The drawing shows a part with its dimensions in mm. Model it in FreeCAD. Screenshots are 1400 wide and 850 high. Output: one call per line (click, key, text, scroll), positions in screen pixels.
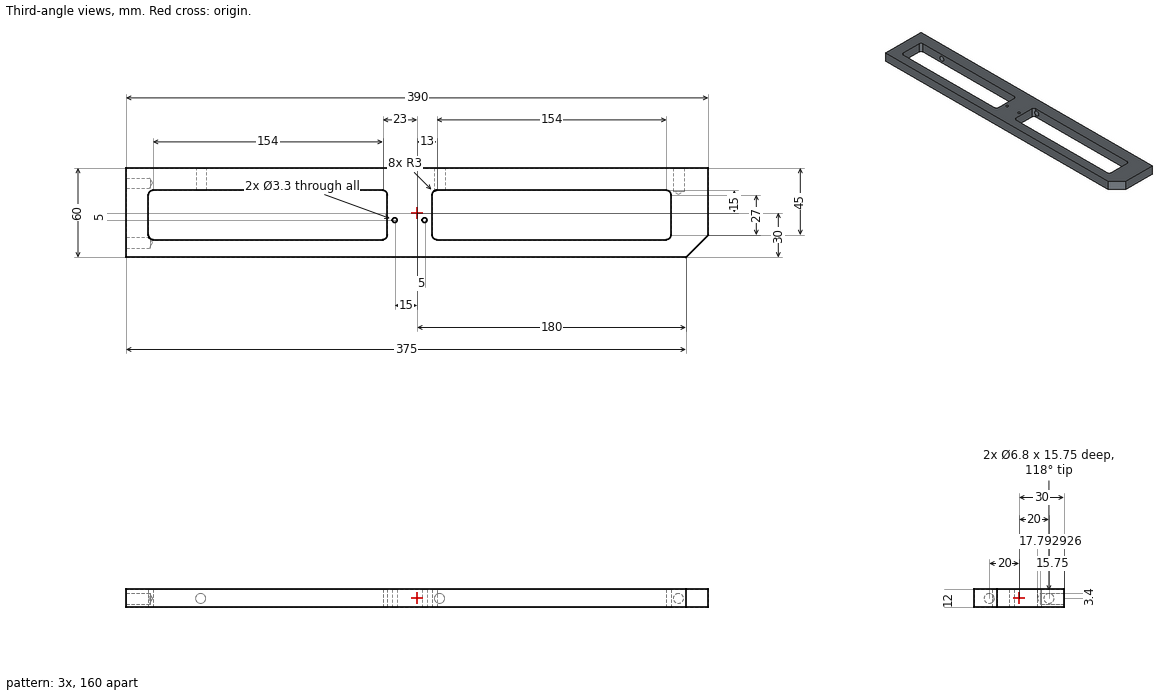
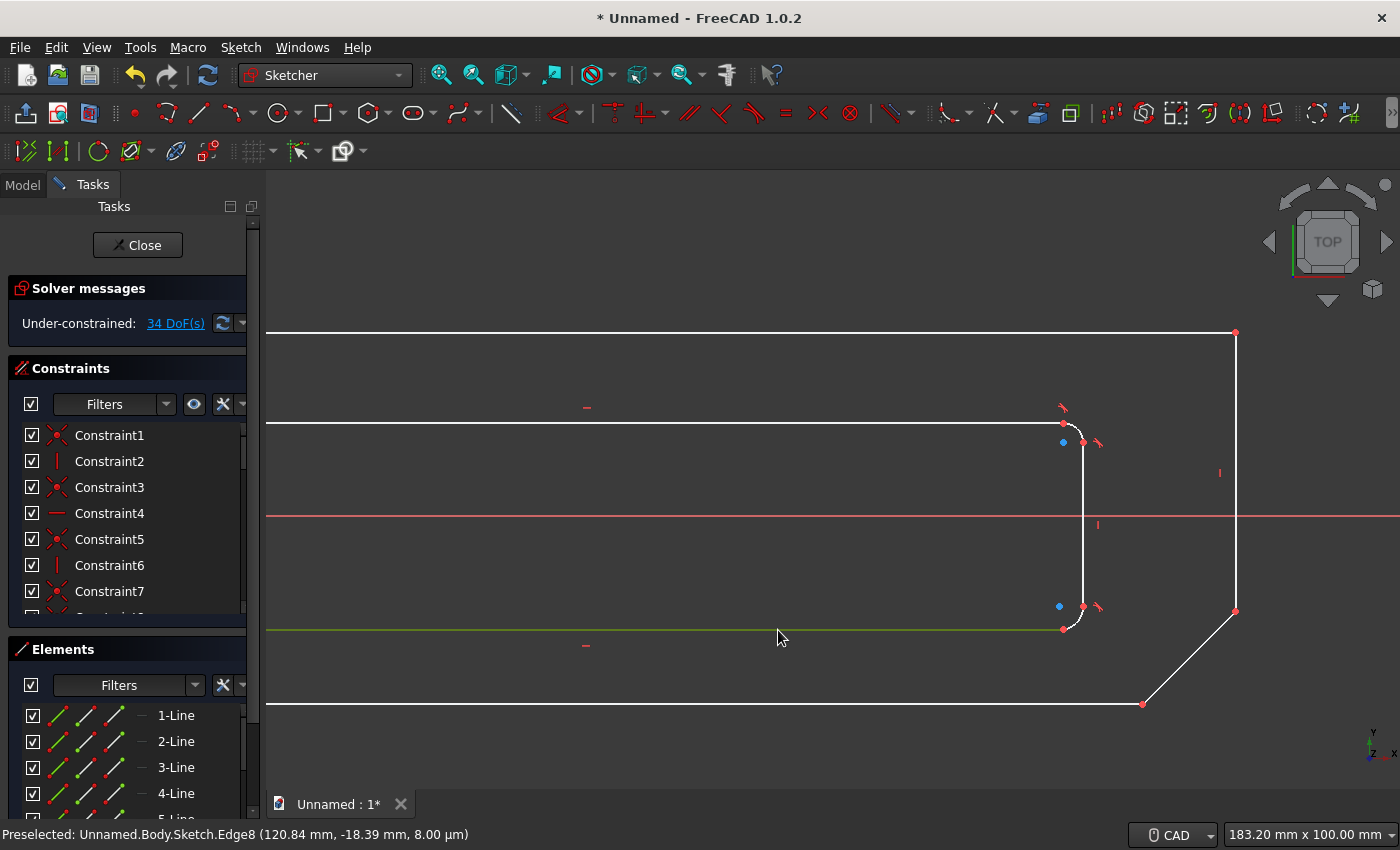
scroll(1073, 626, up, 2)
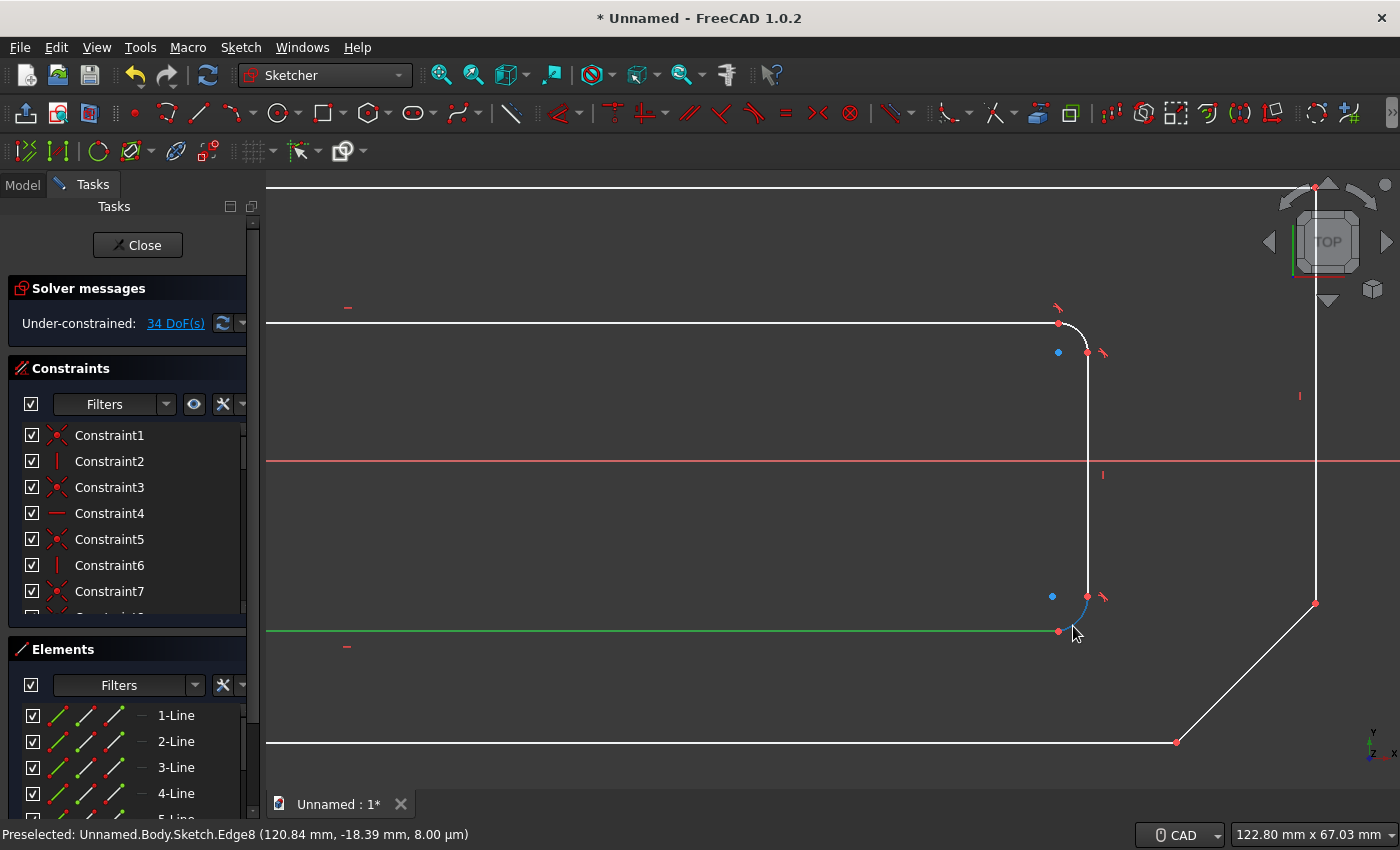
click(1072, 626)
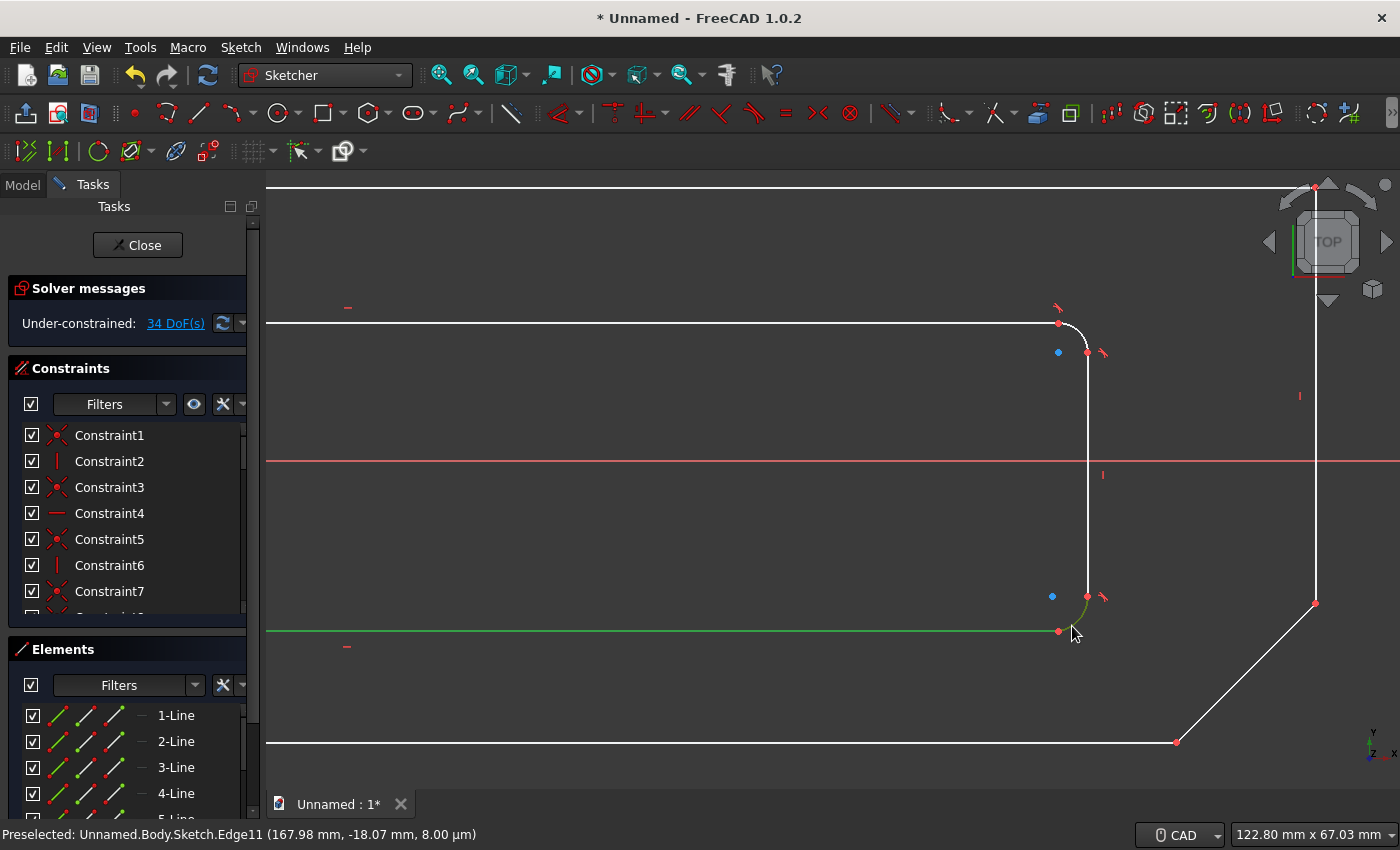
click(754, 114)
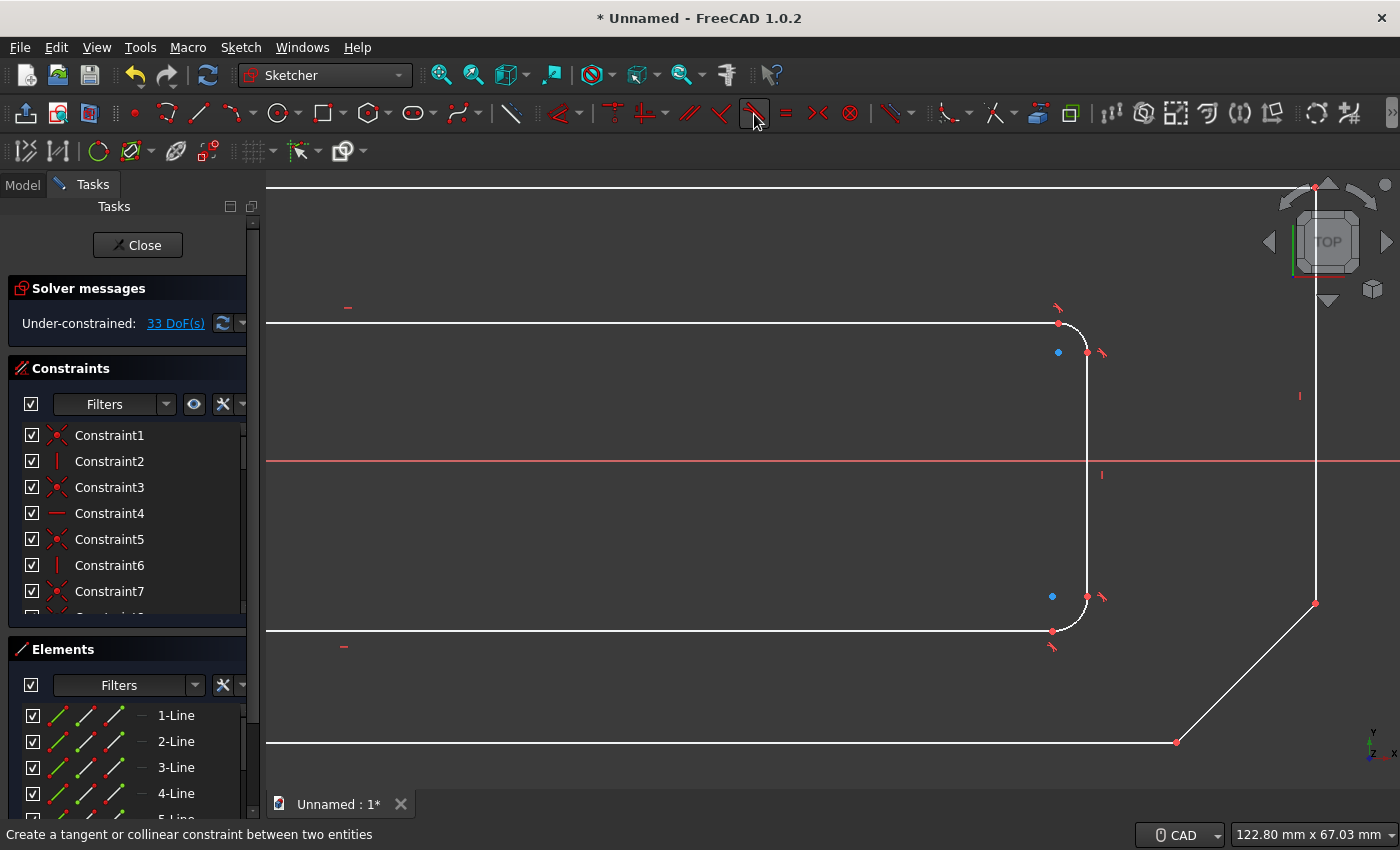
scroll(1080, 484, down, 8)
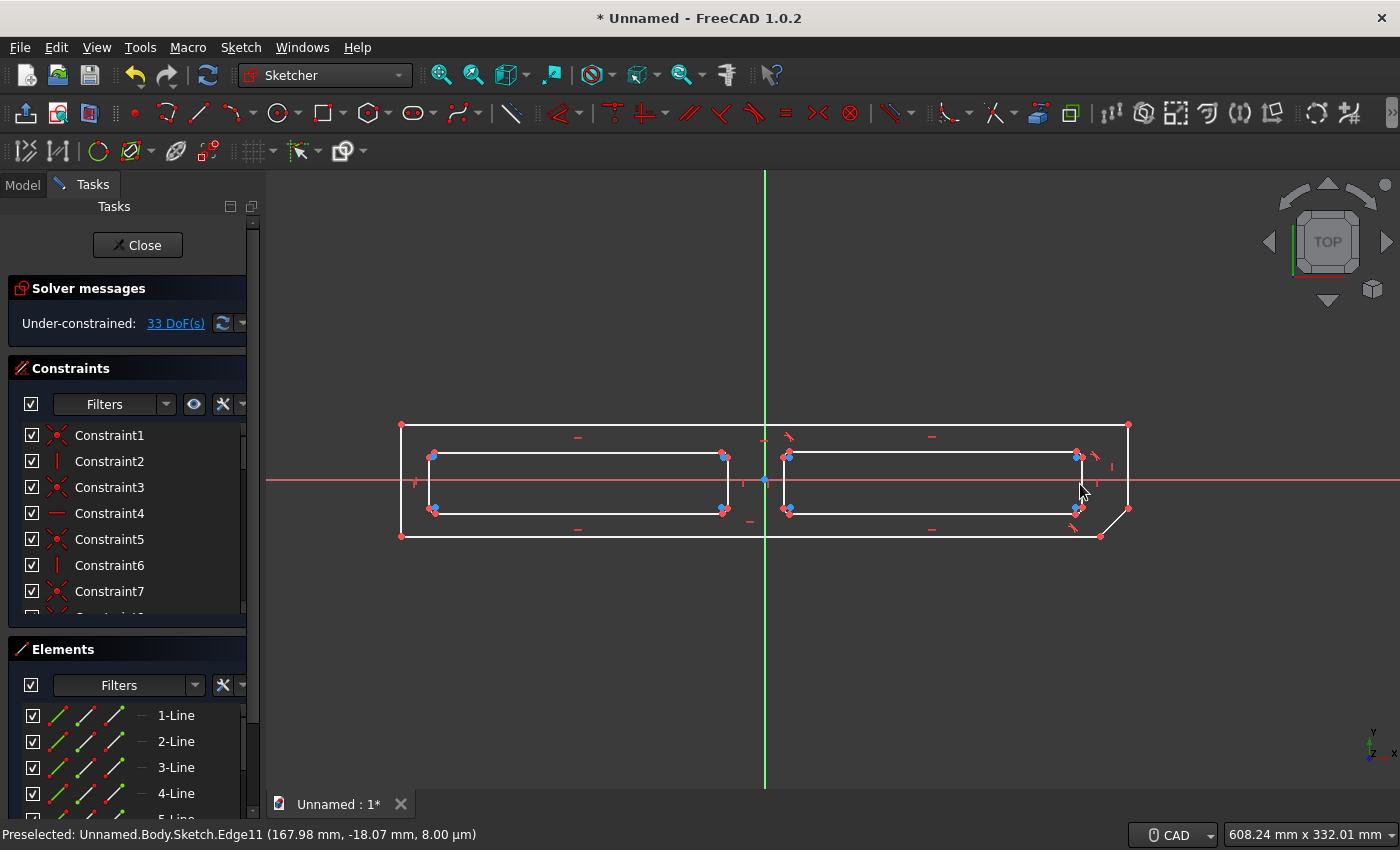
click(989, 514)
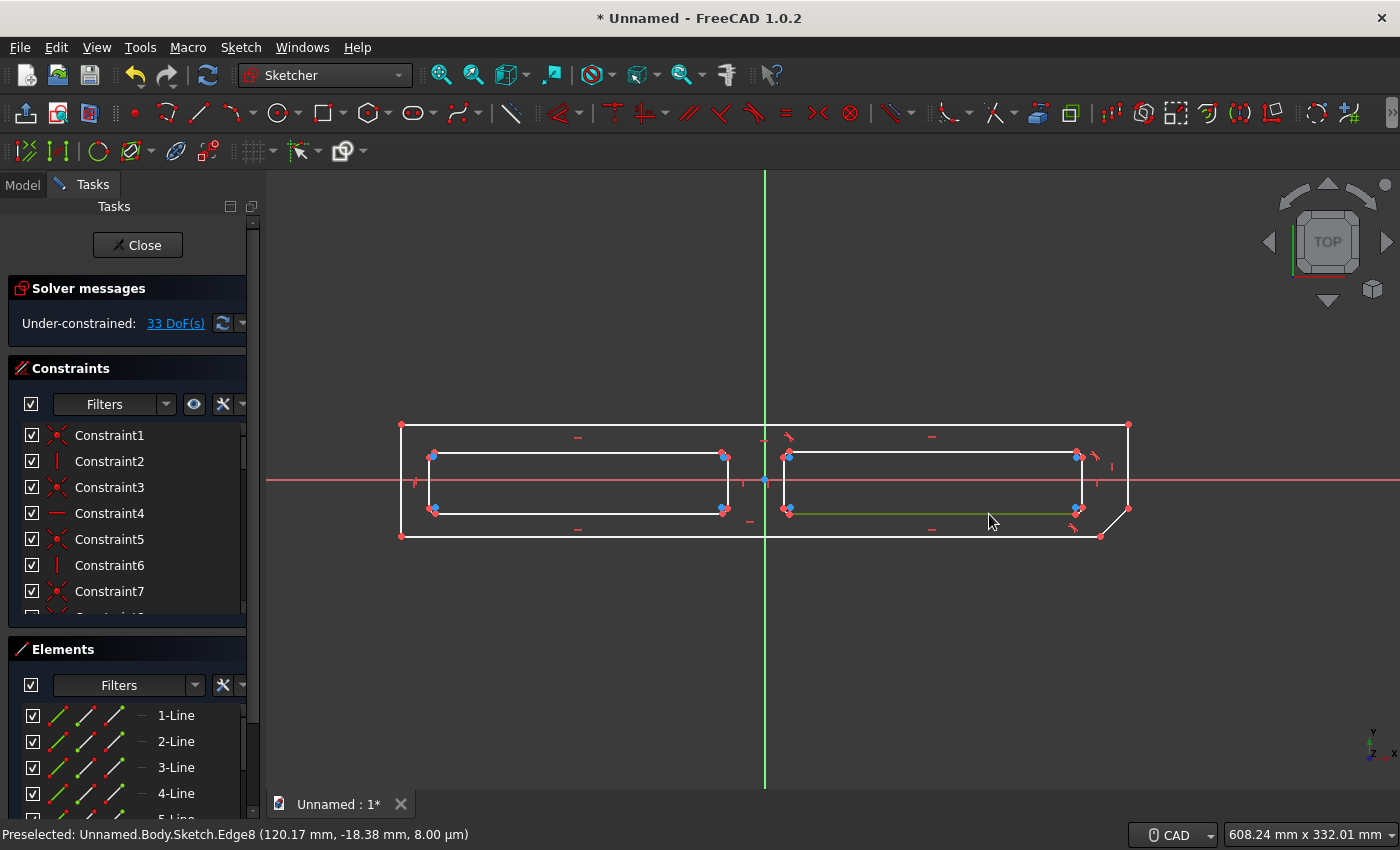
scroll(785, 512, up, 6)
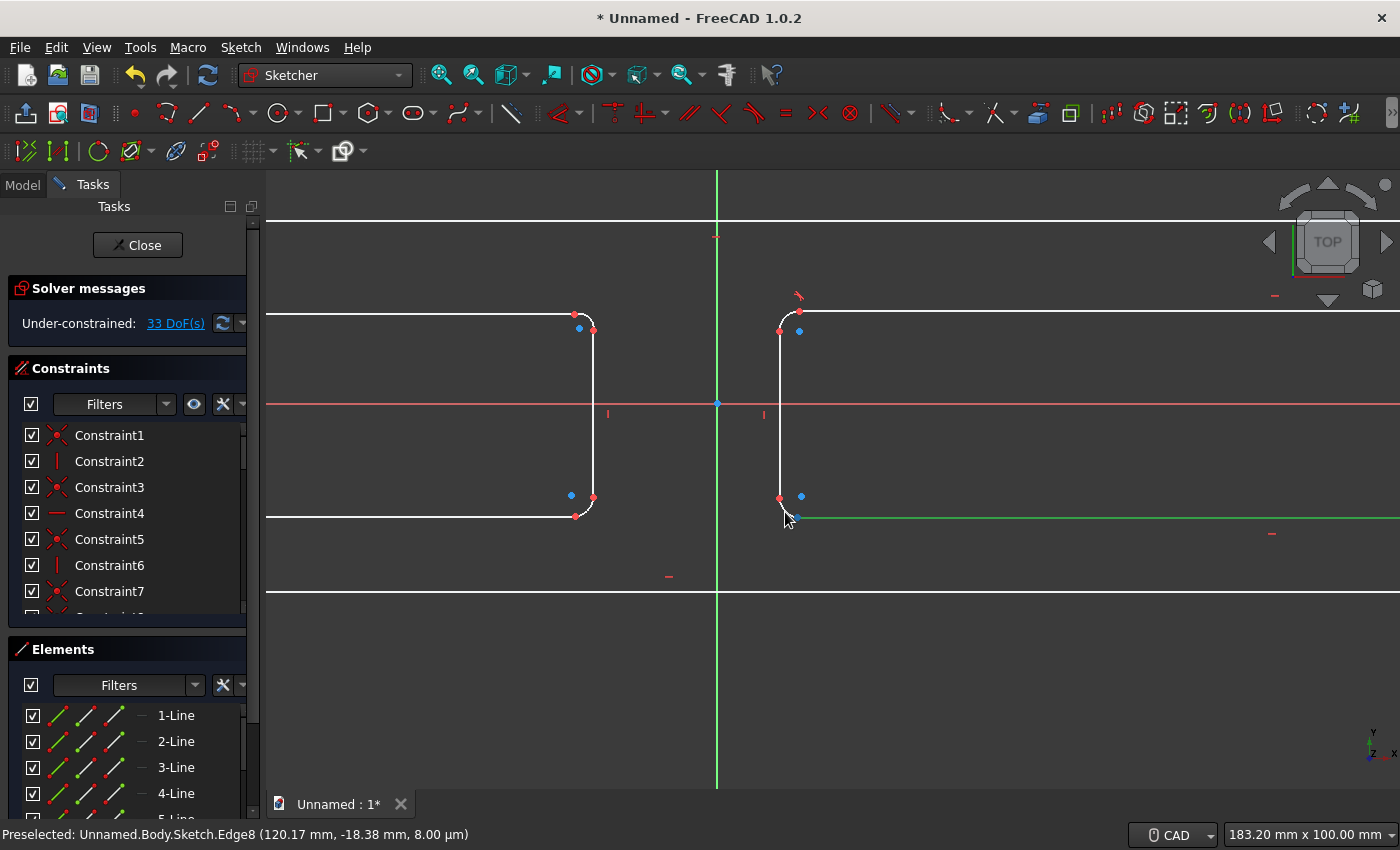
click(785, 511)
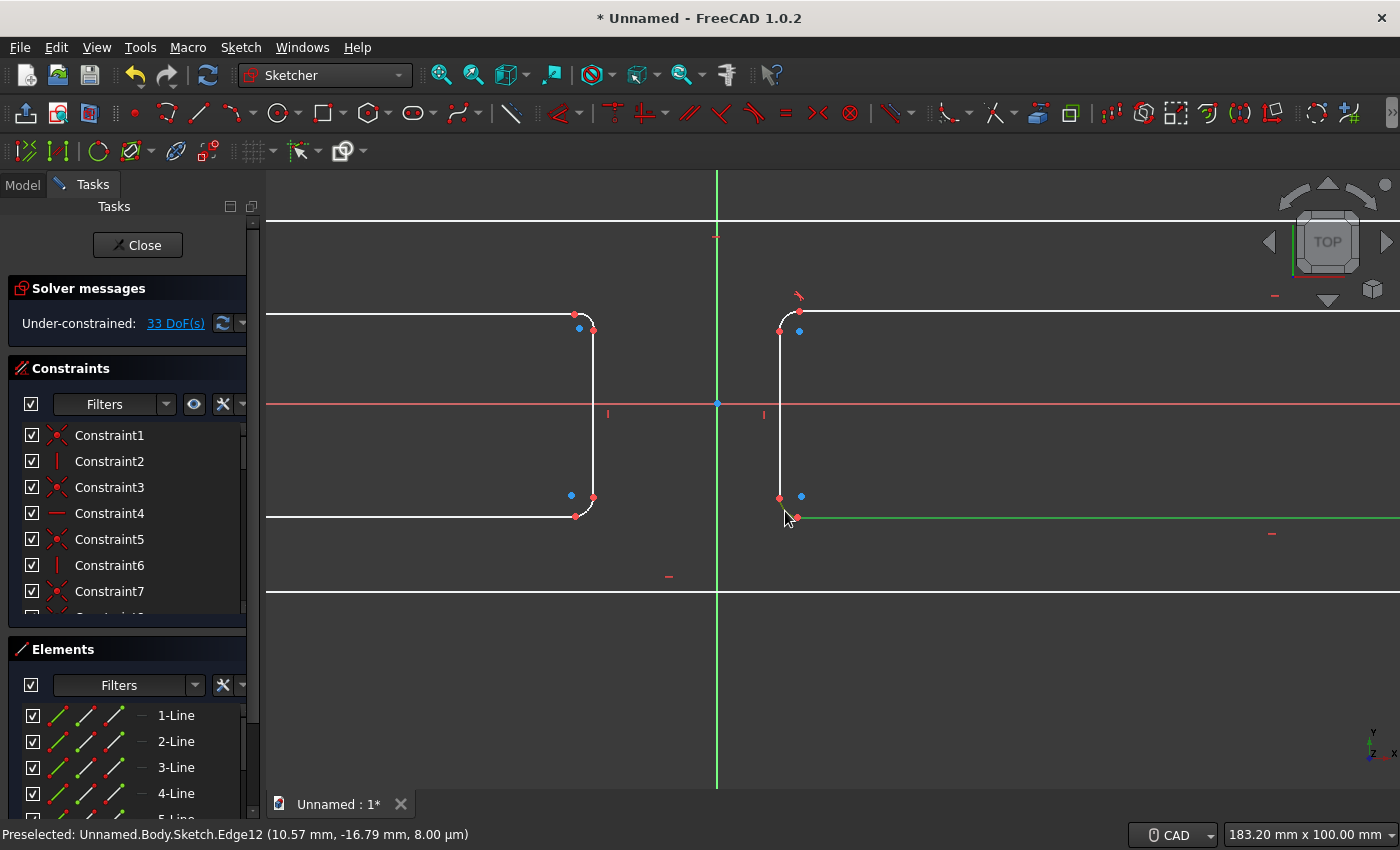
click(754, 114)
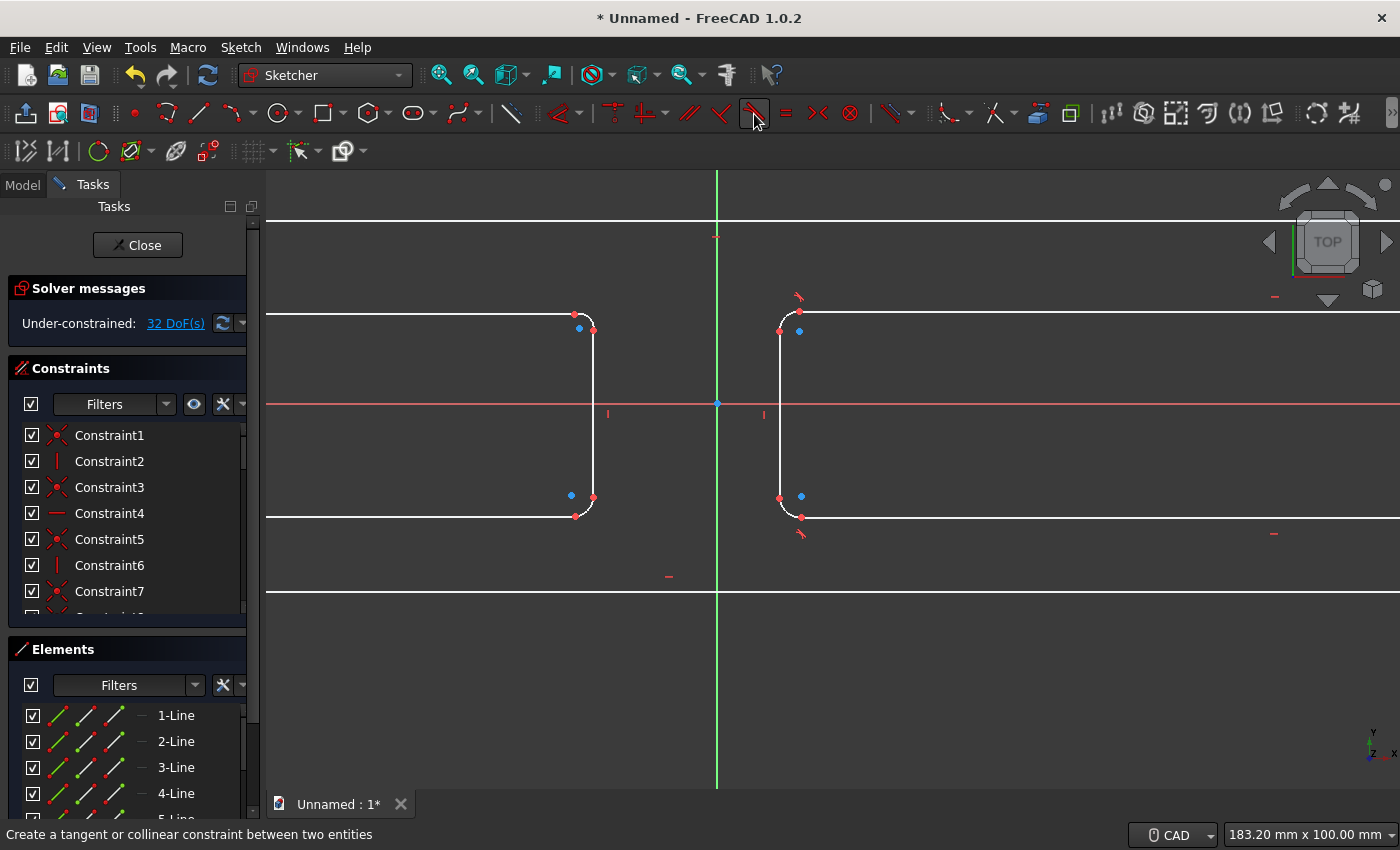
click(780, 448)